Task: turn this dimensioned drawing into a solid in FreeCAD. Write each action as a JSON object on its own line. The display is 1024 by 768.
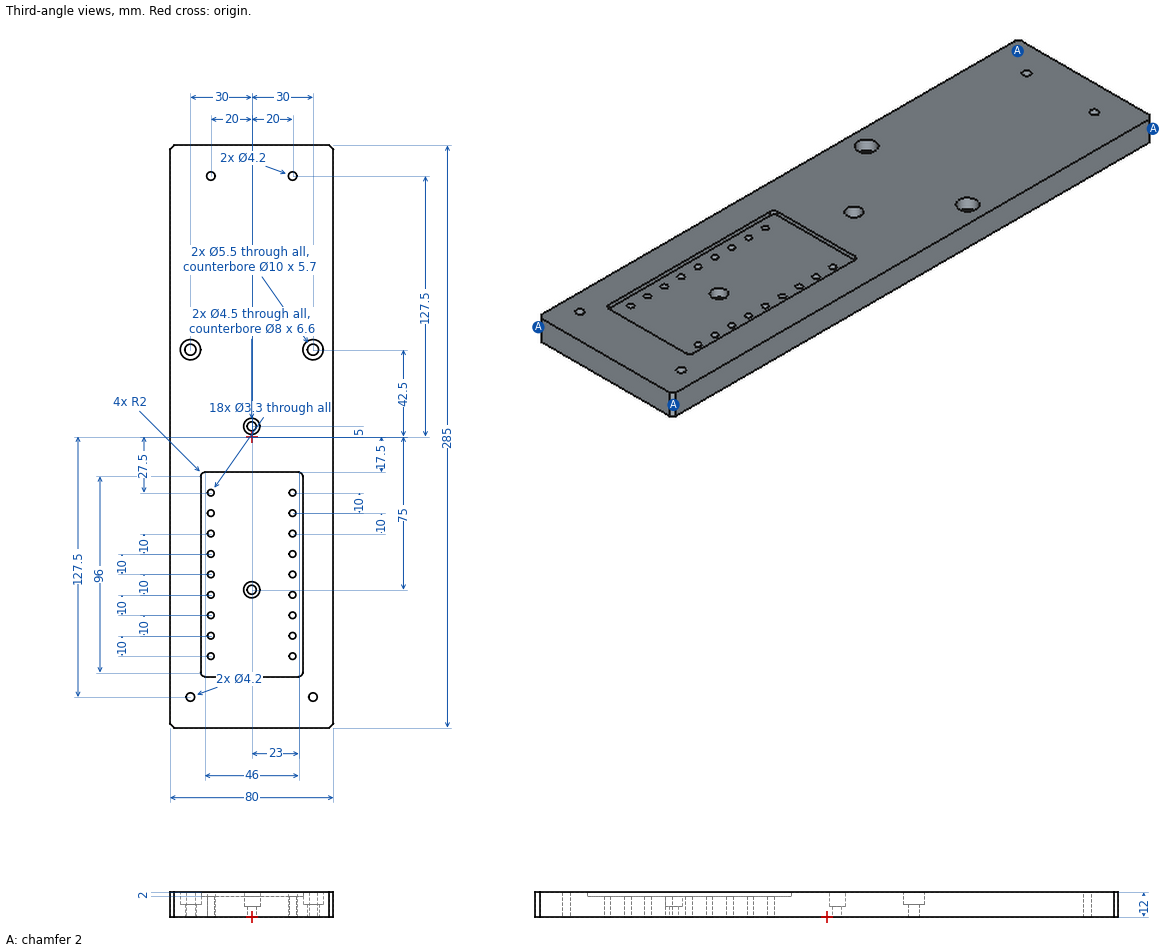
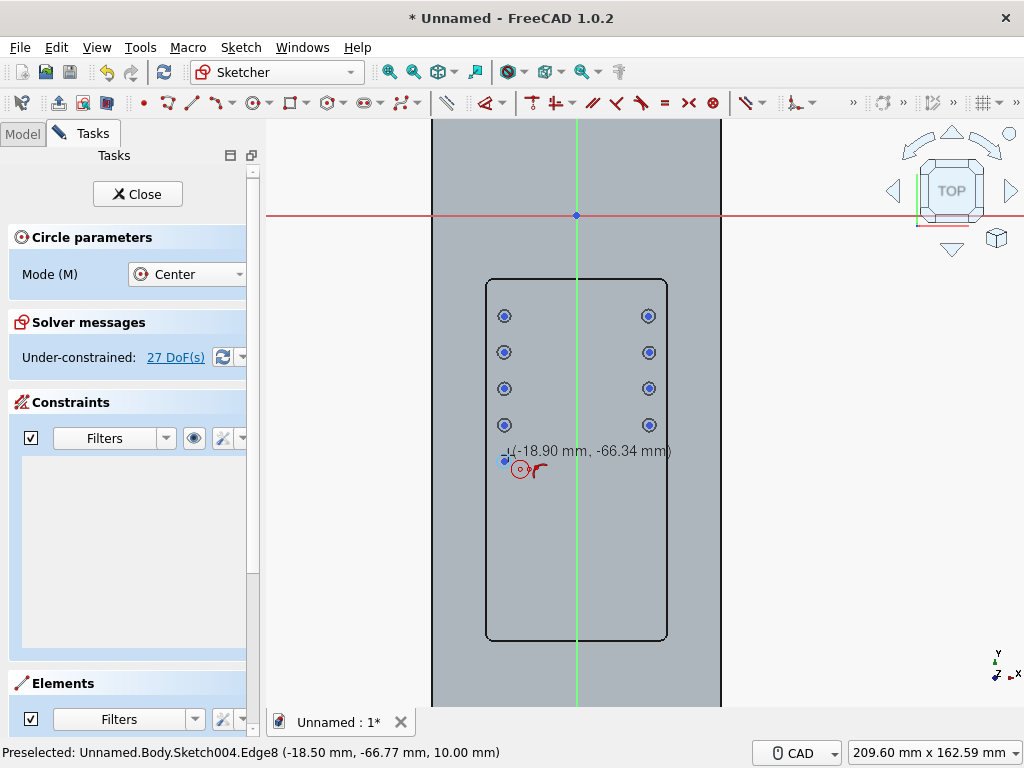
{"action": "scroll", "coordinate": [649, 460], "scroll_direction": "up", "scroll_amount": 7}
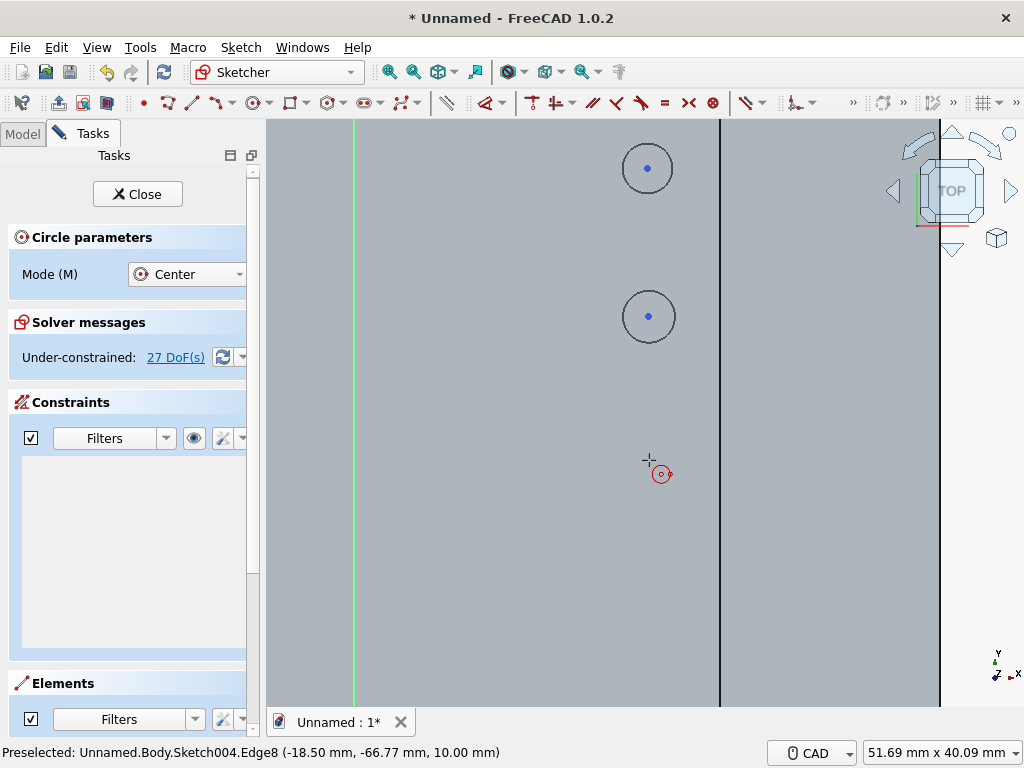
{"action": "scroll", "coordinate": [649, 460], "scroll_direction": "down", "scroll_amount": 7}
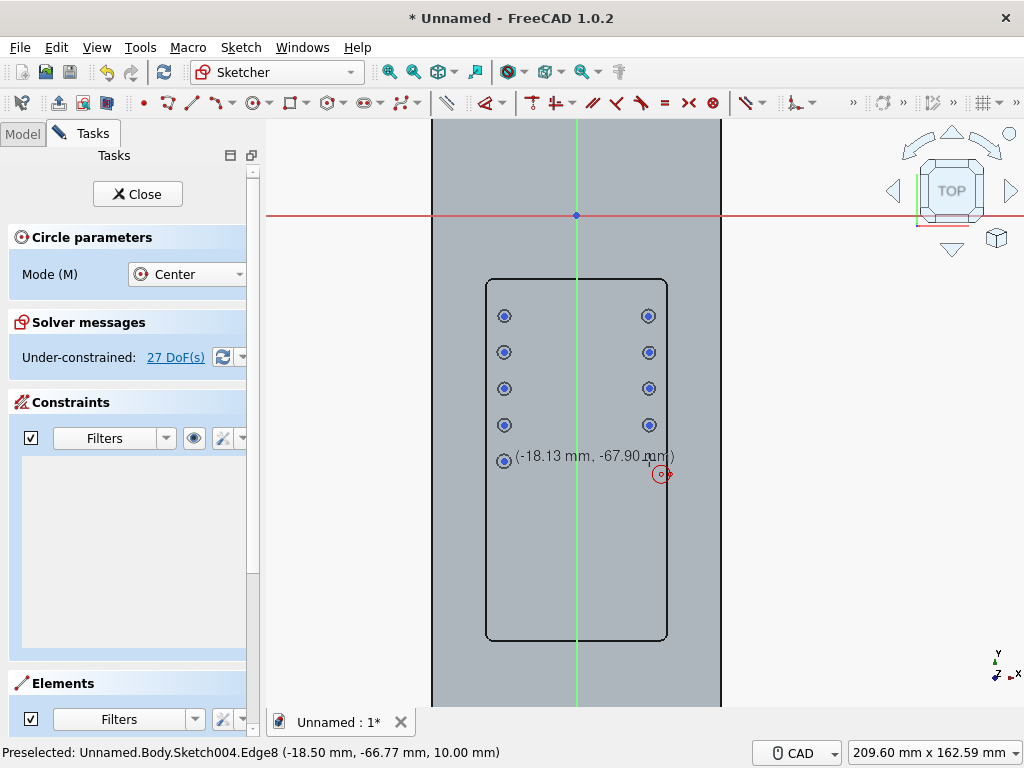
{"action": "left_click", "coordinate": [649, 460]}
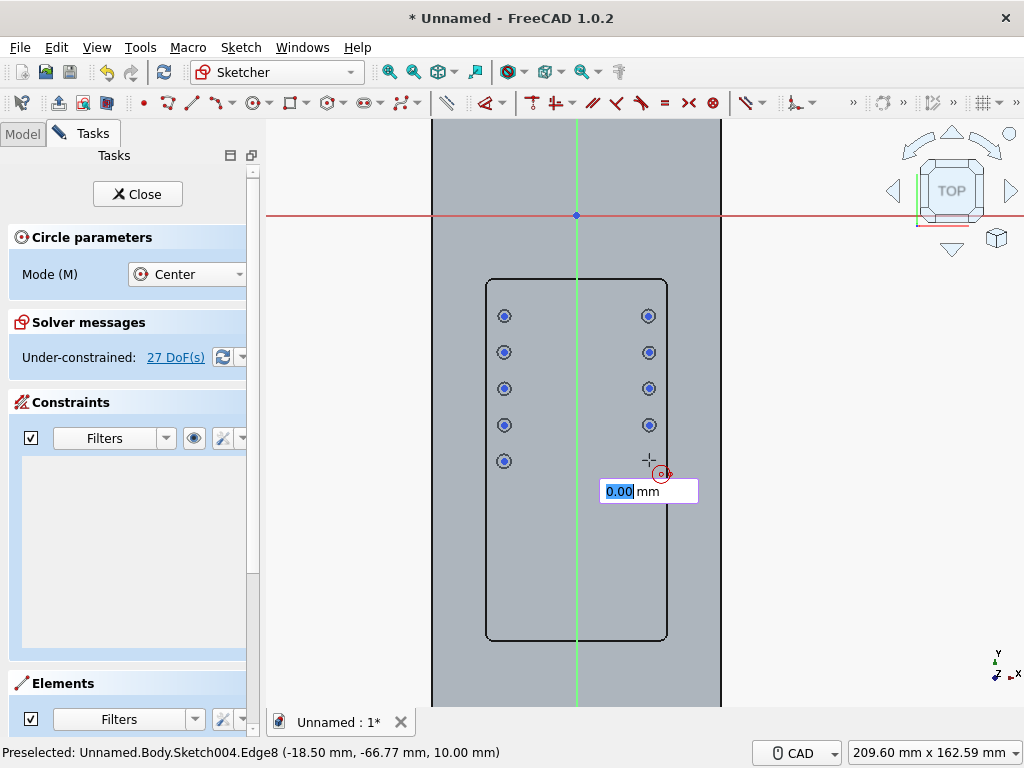
{"action": "scroll", "coordinate": [653, 456], "scroll_direction": "up", "scroll_amount": 5}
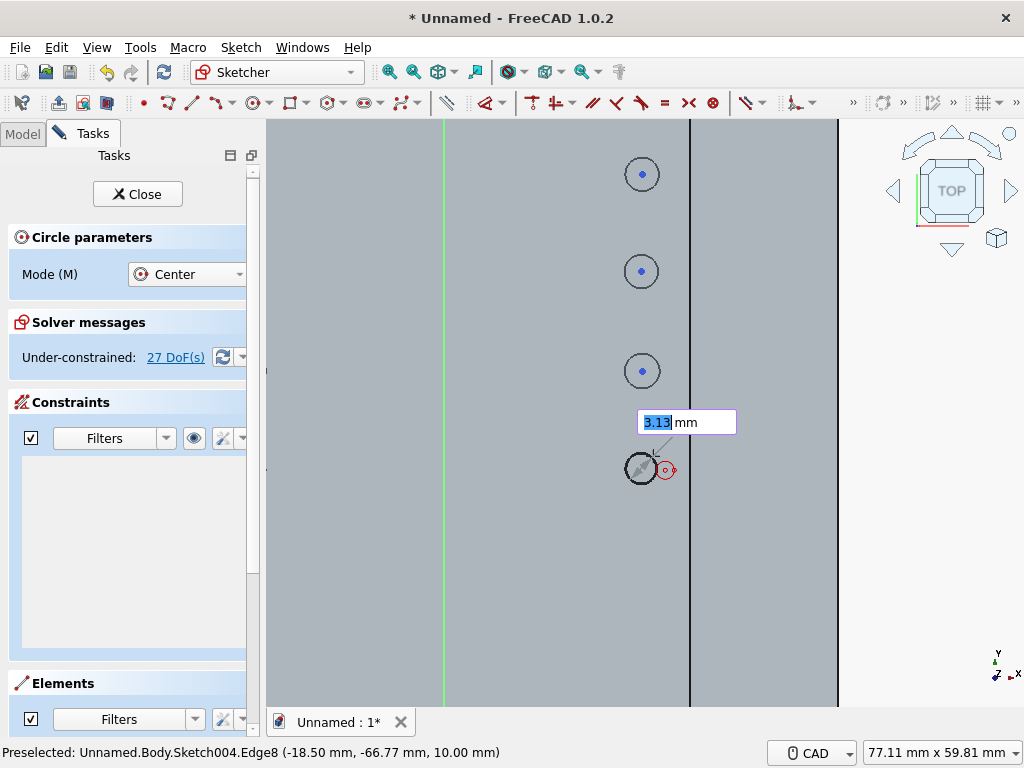
{"action": "left_click", "coordinate": [652, 454]}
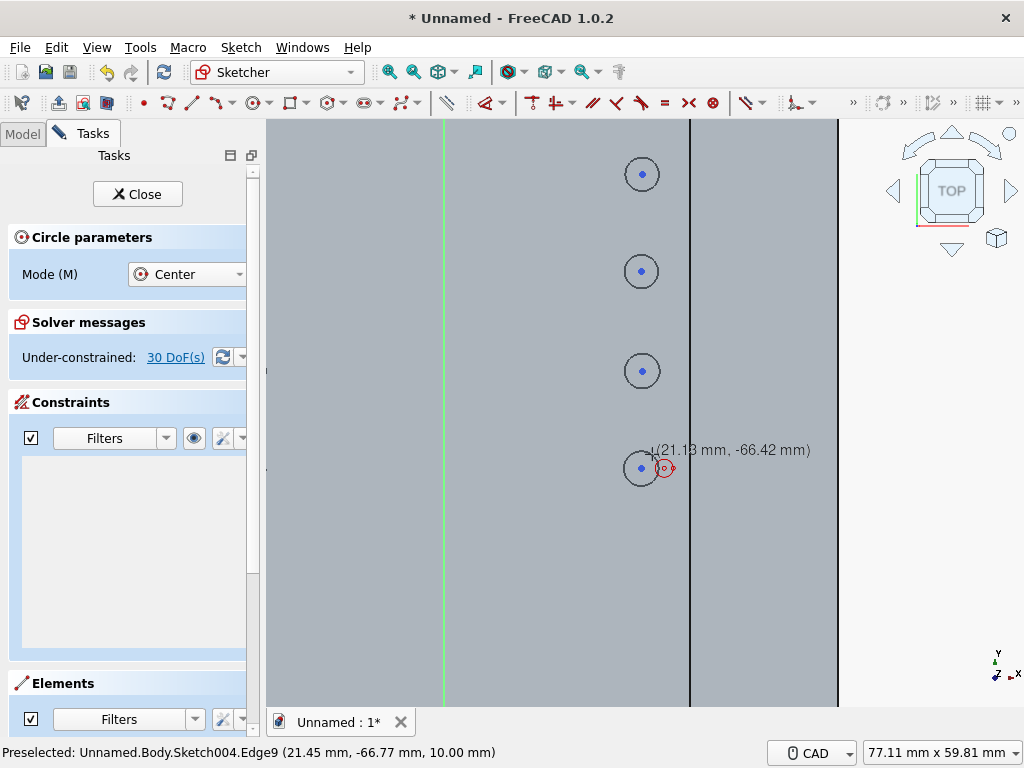
{"action": "scroll", "coordinate": [653, 456], "scroll_direction": "down", "scroll_amount": 5}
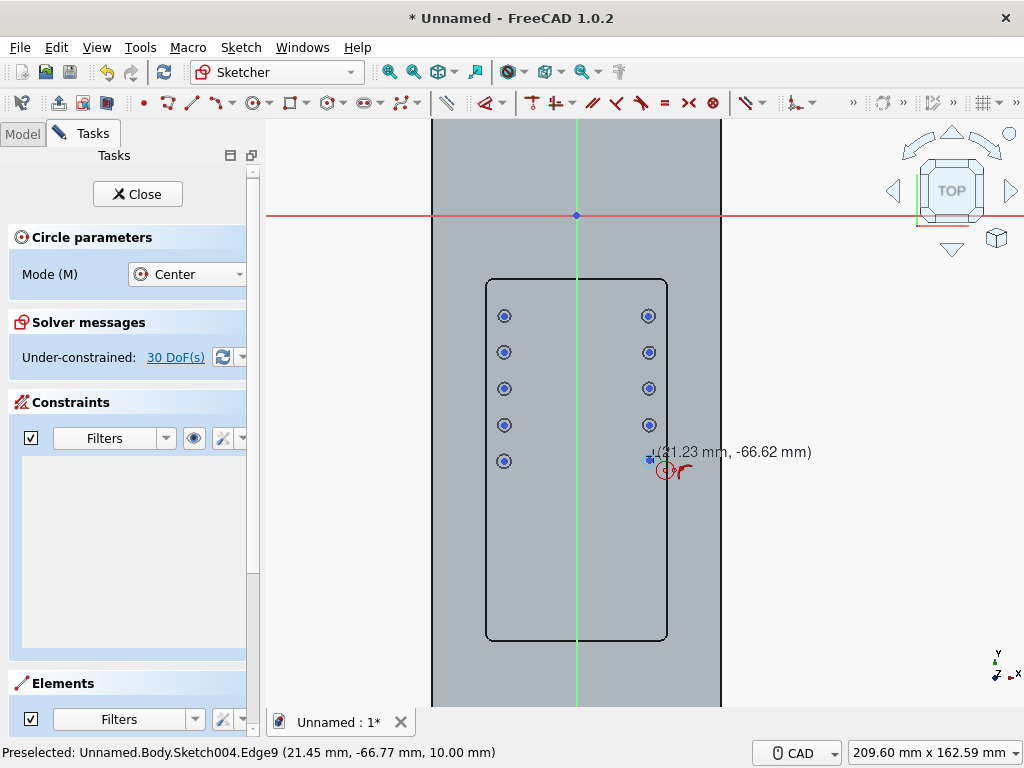
{"action": "scroll", "coordinate": [504, 496], "scroll_direction": "up", "scroll_amount": 7}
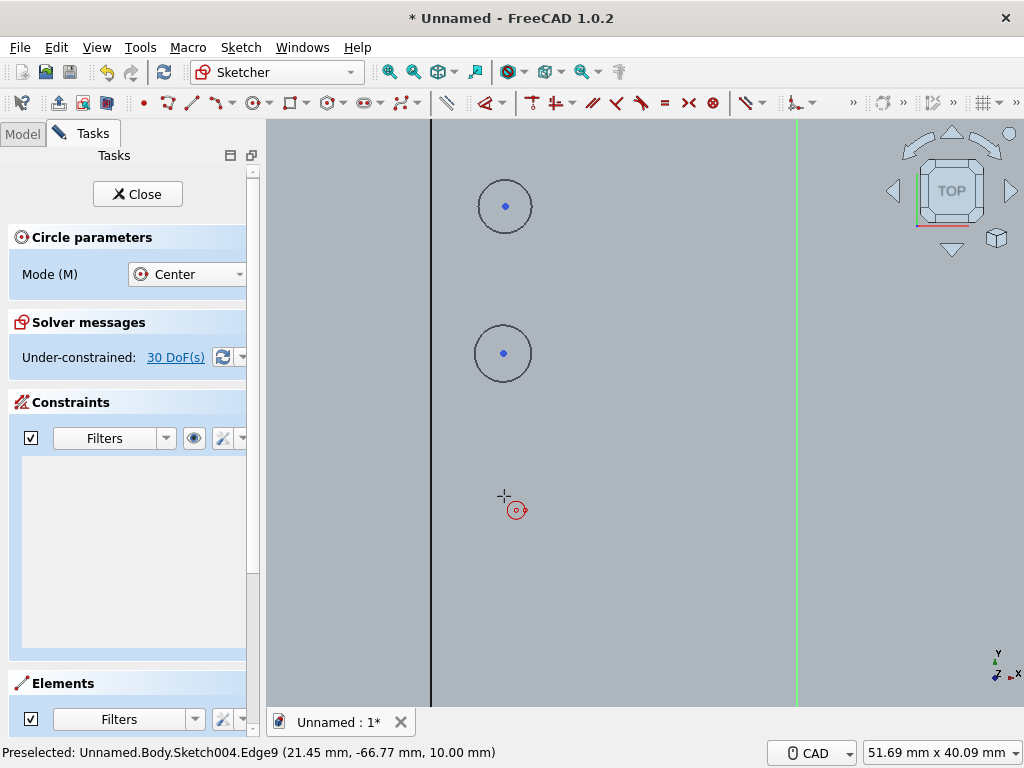
{"action": "scroll", "coordinate": [504, 496], "scroll_direction": "down", "scroll_amount": 7}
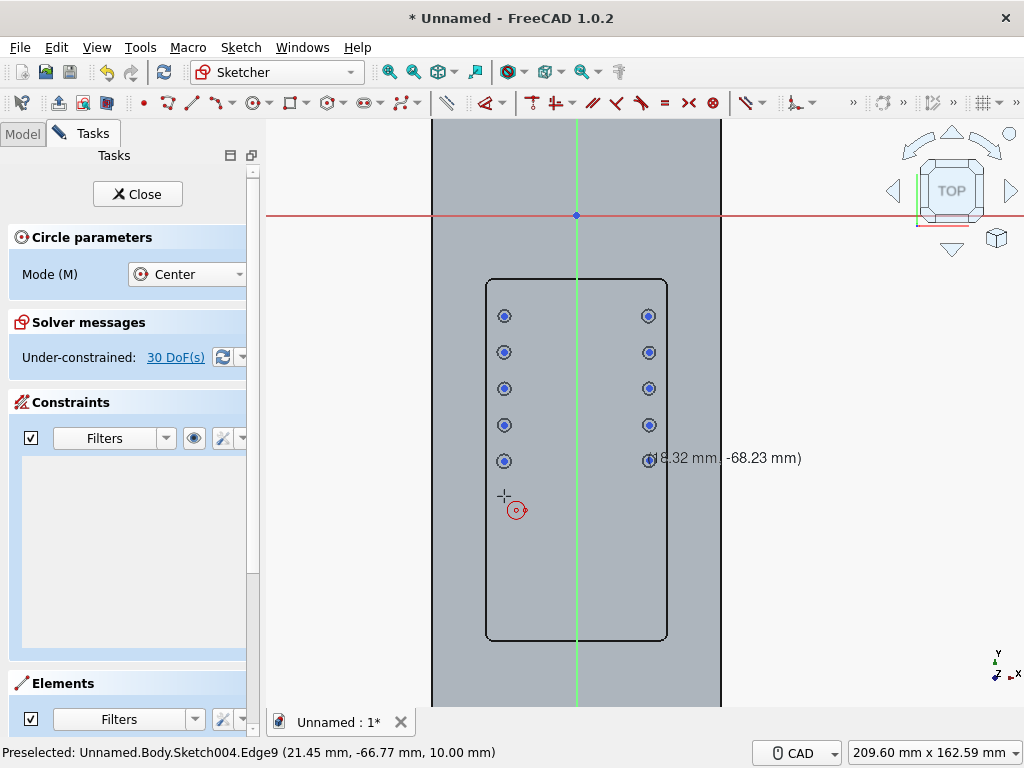
{"action": "left_click", "coordinate": [504, 496]}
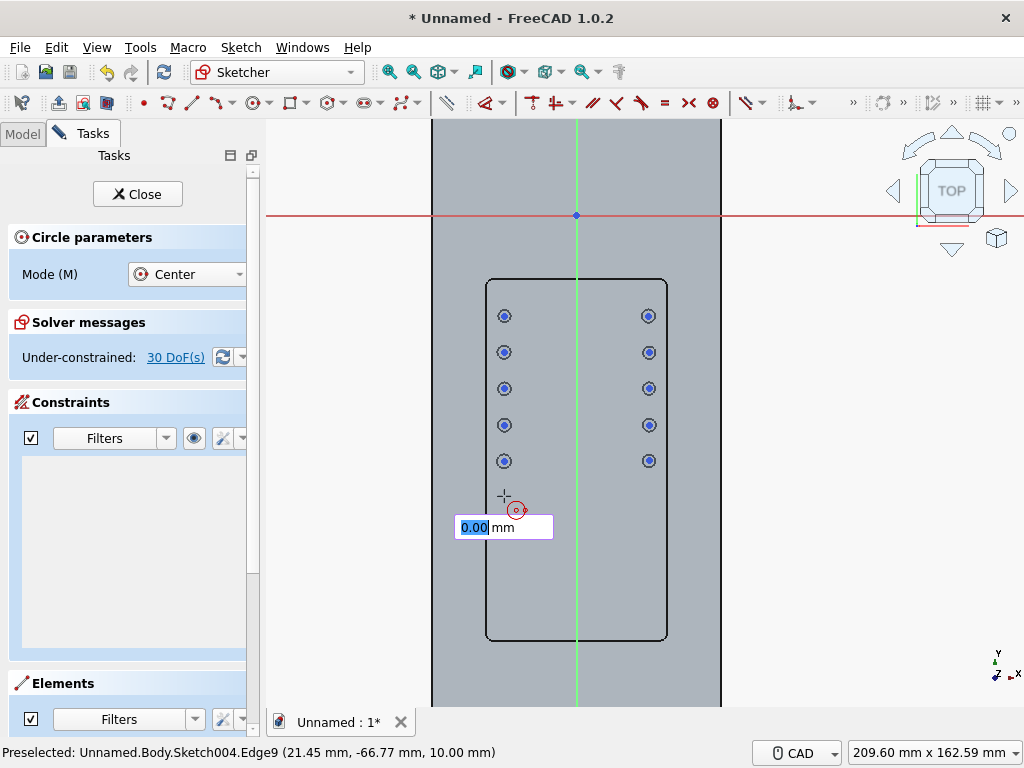
{"action": "scroll", "coordinate": [508, 492], "scroll_direction": "up", "scroll_amount": 5}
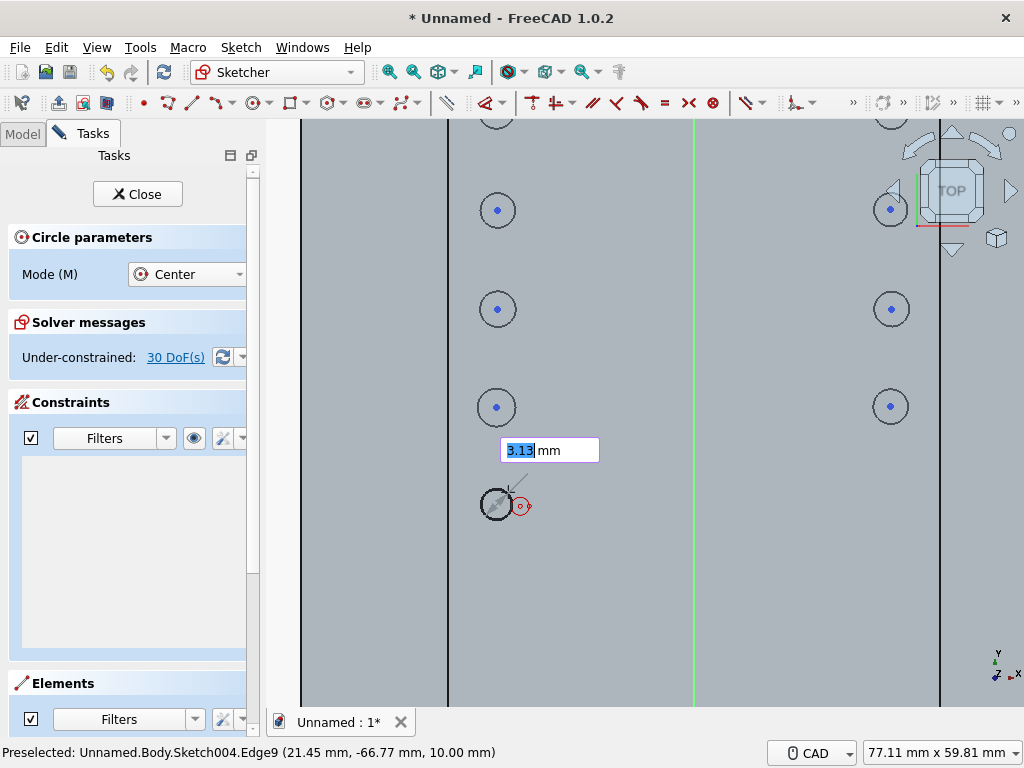
{"action": "left_click", "coordinate": [509, 491]}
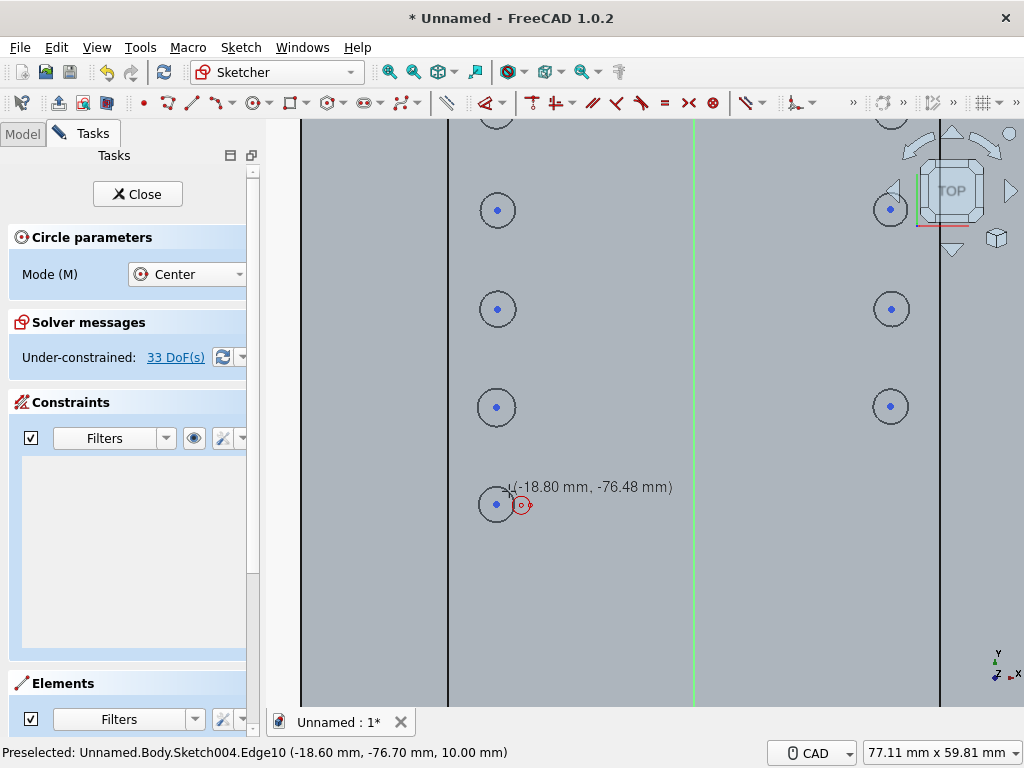
{"action": "scroll", "coordinate": [508, 492], "scroll_direction": "down", "scroll_amount": 5}